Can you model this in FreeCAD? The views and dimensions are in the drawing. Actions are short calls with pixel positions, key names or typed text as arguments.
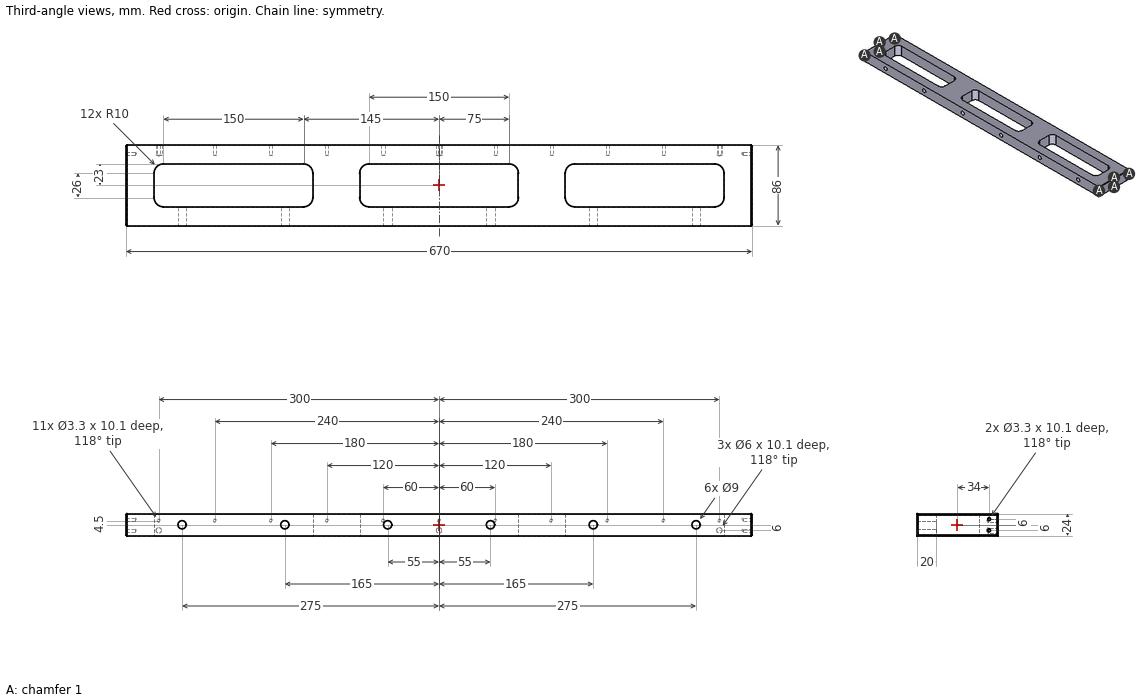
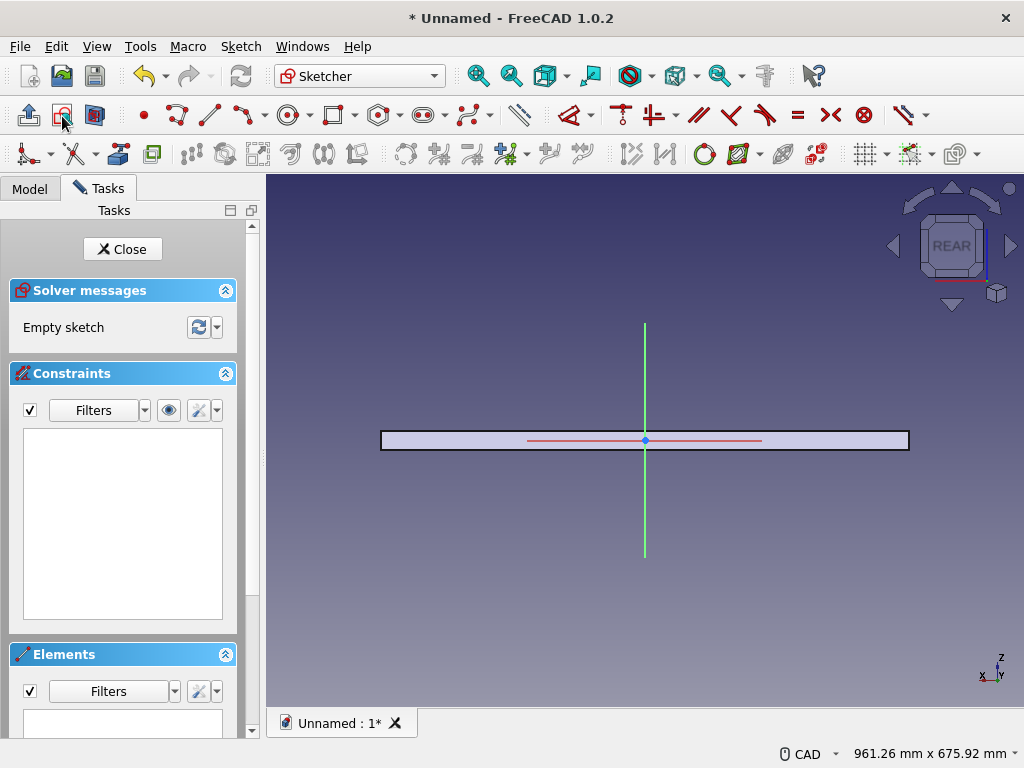
scroll(294, 451, down, 1)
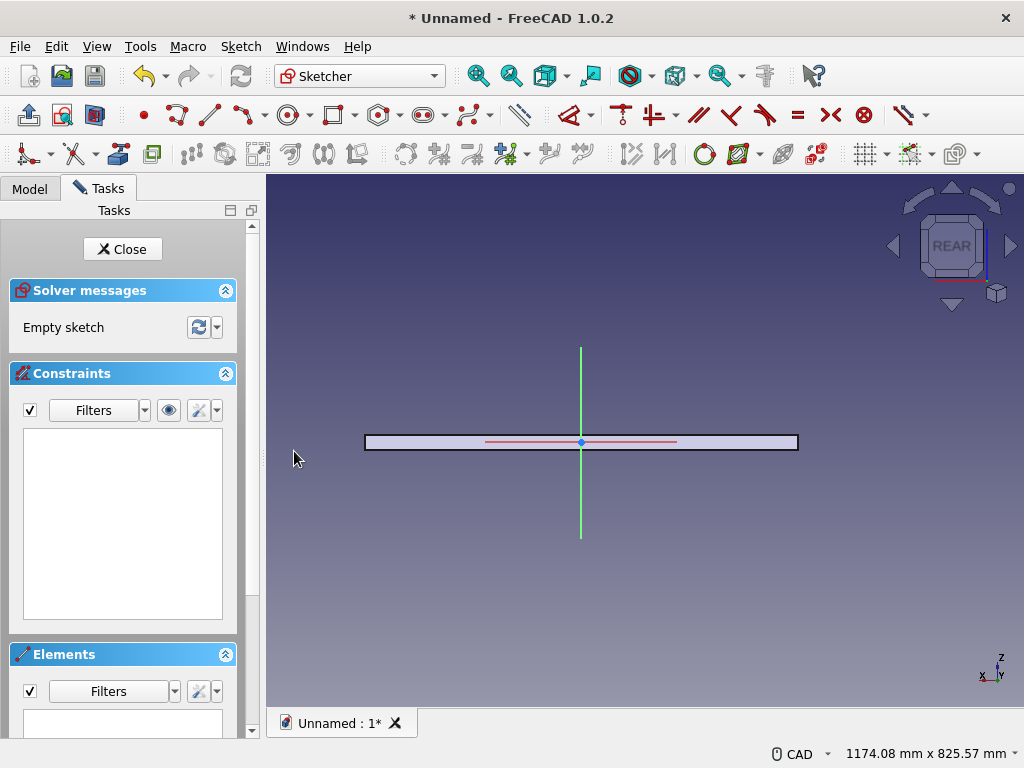
key(g)
key(c)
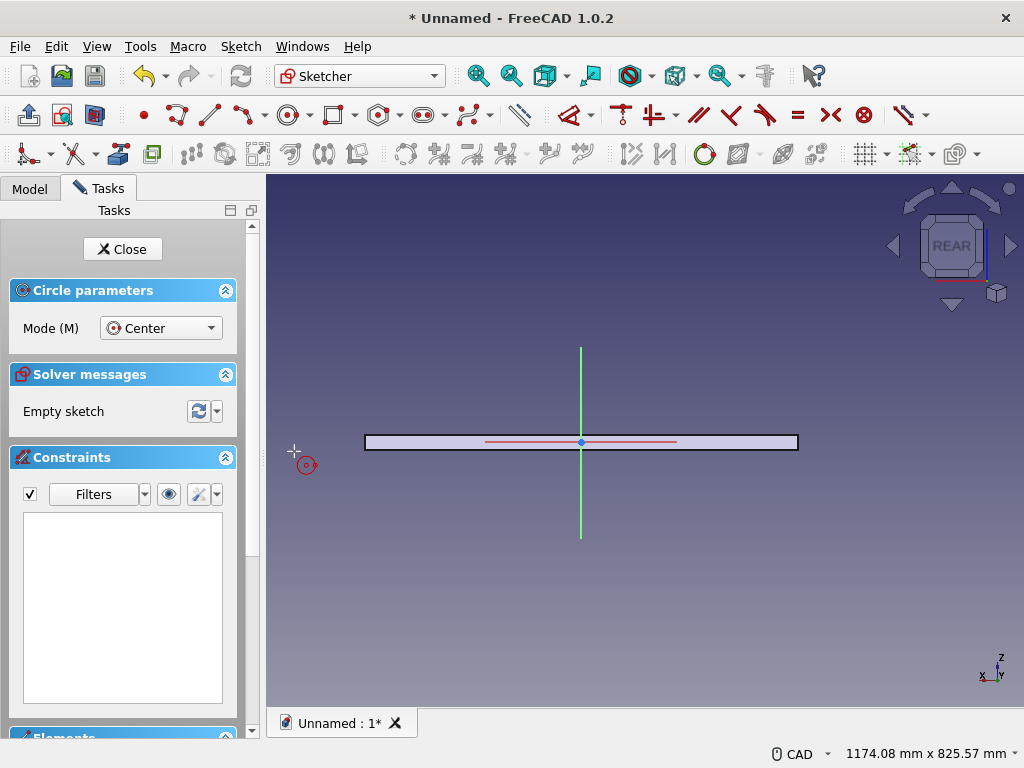
scroll(775, 440, up, 16)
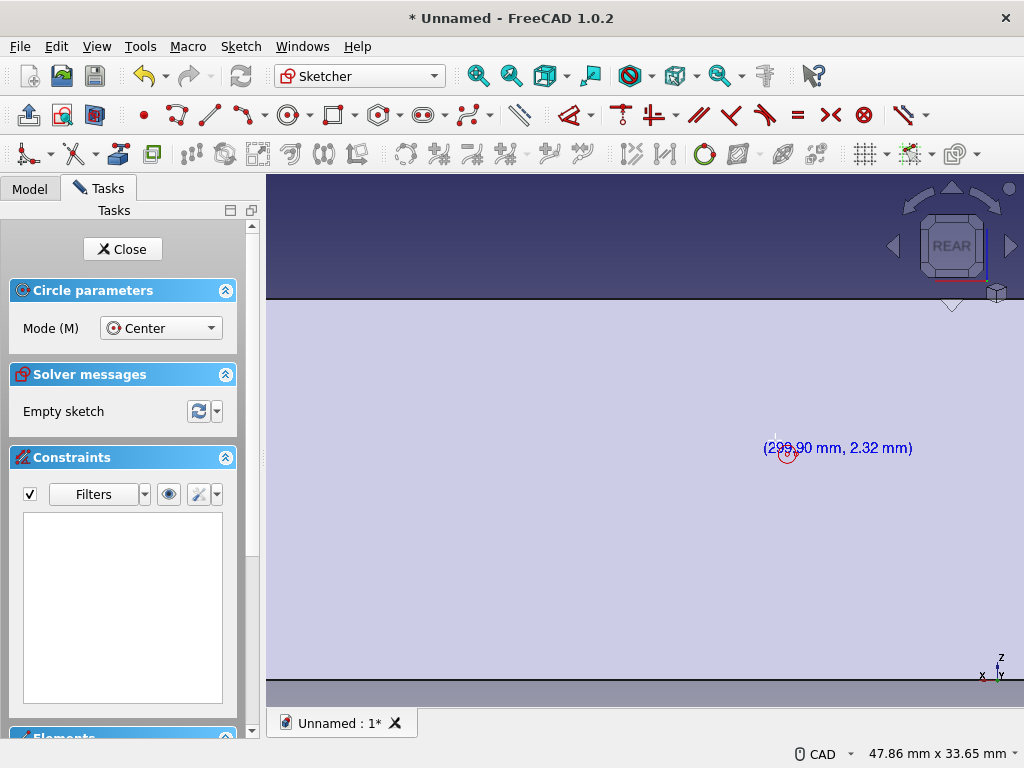
scroll(816, 440, down, 15)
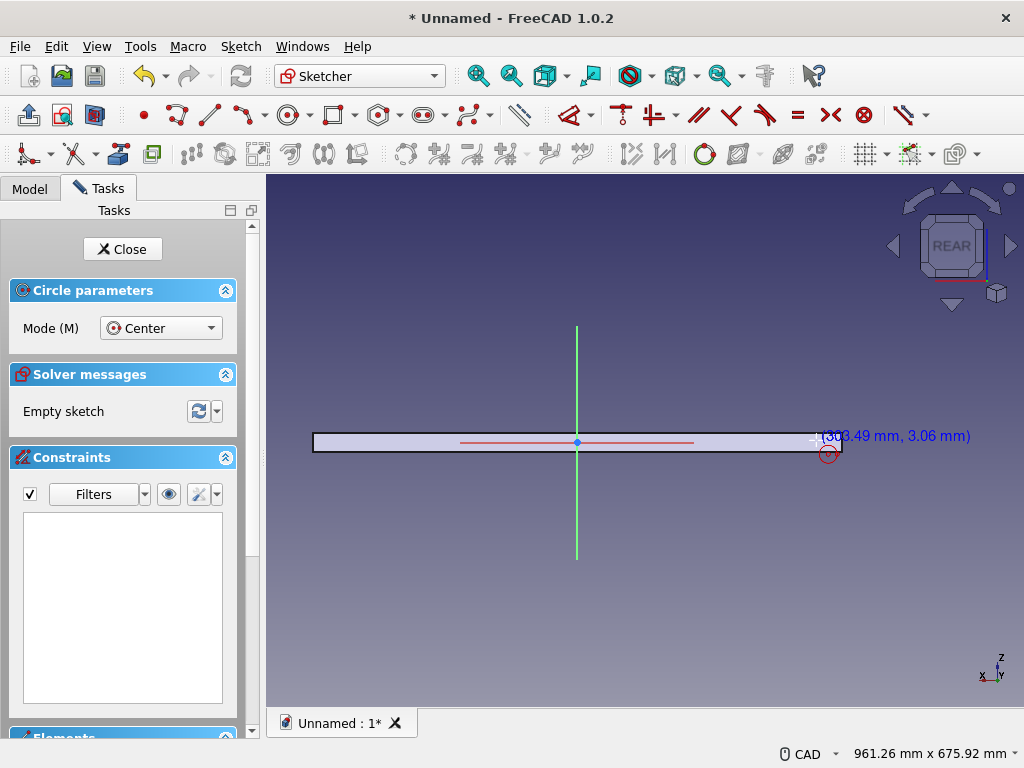
scroll(814, 439, up, 8)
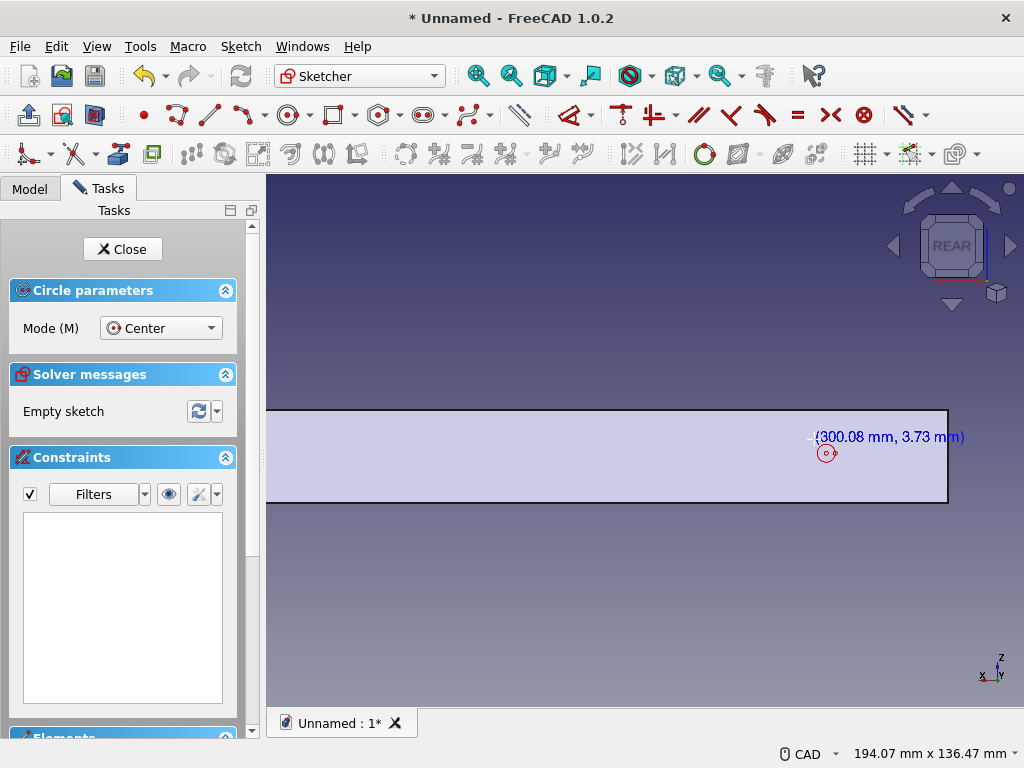
click(811, 439)
move(815, 434)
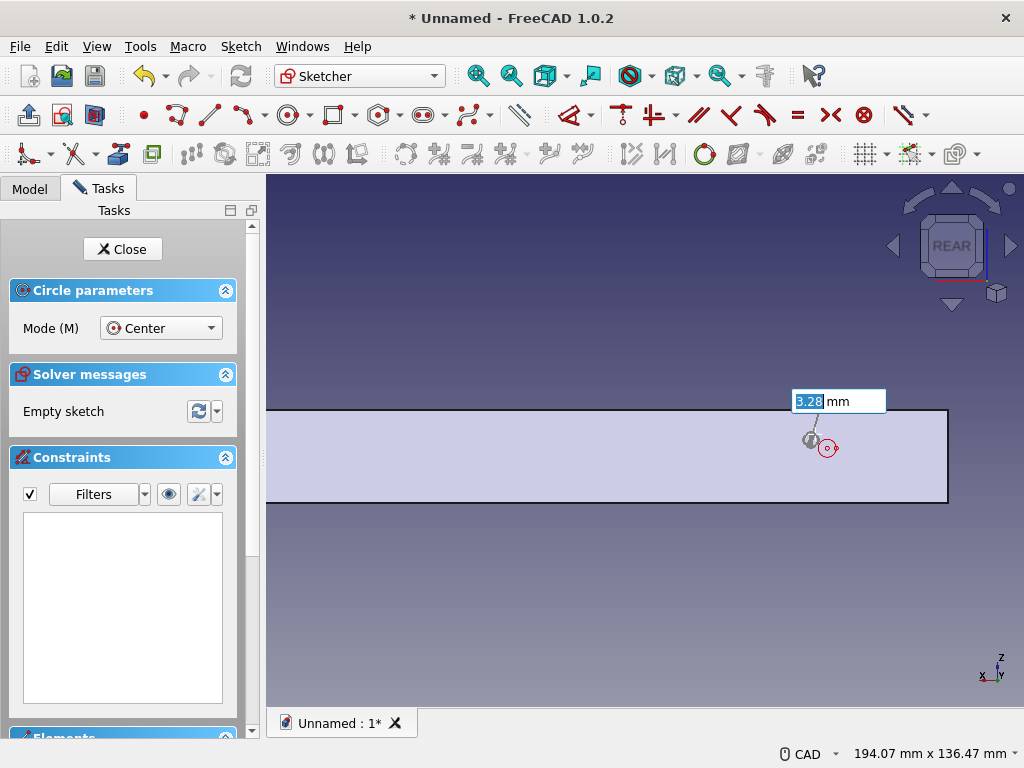
text(3.3)
key(Return)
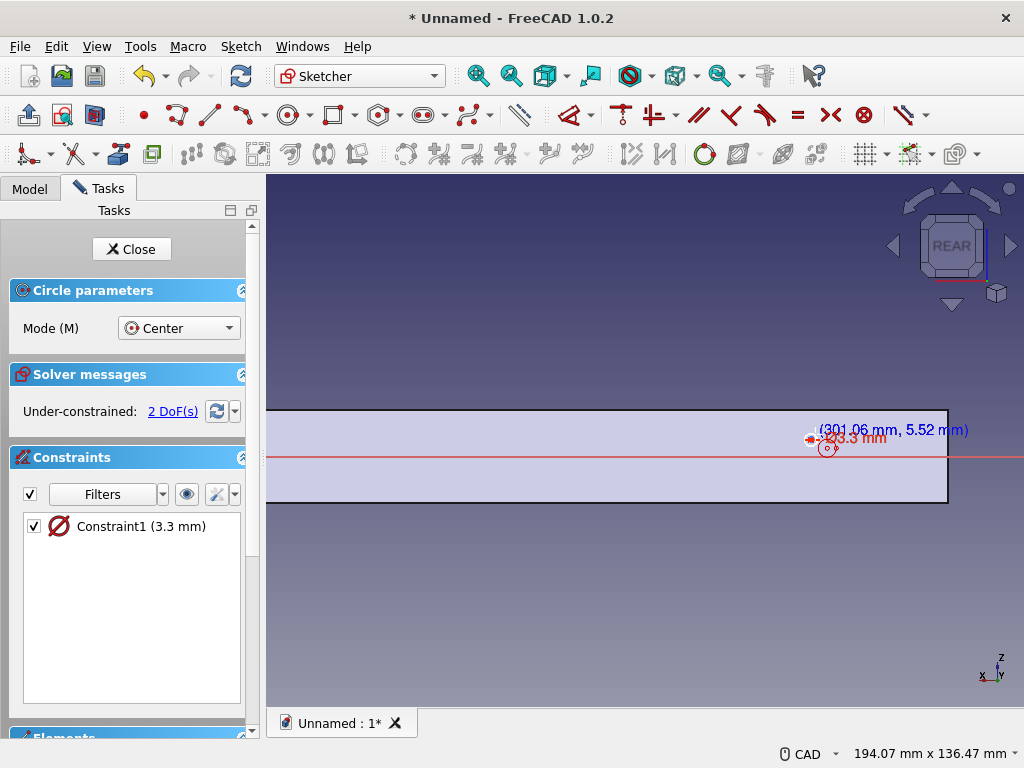
scroll(576, 439, up, 7)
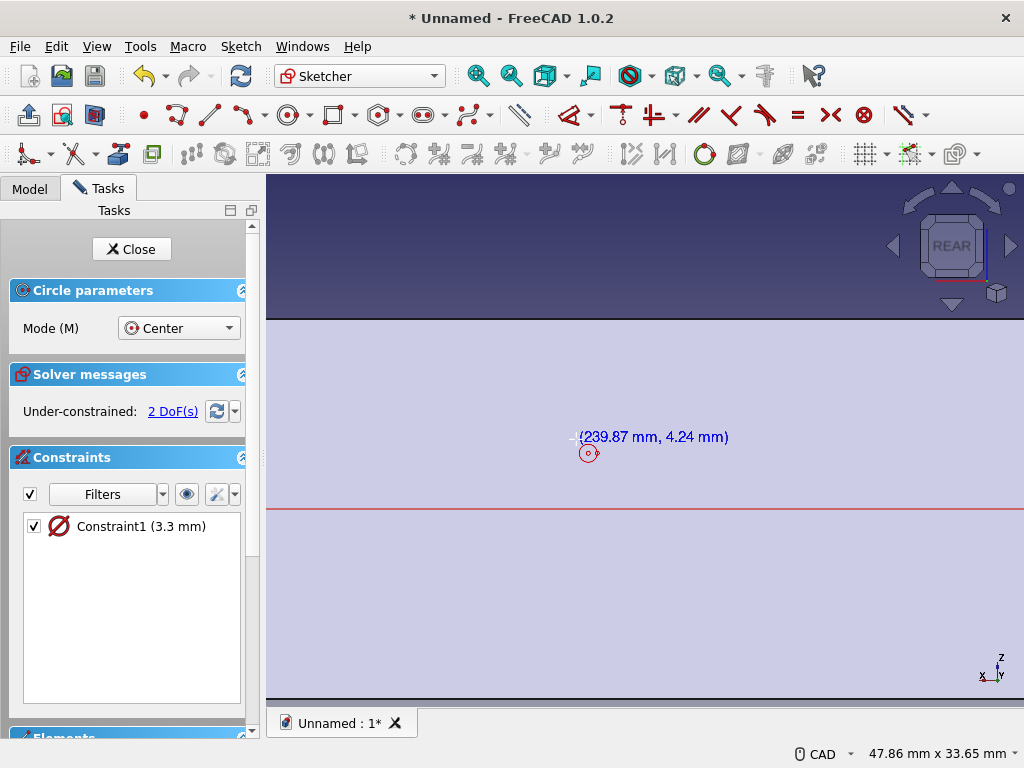
scroll(776, 439, down, 15)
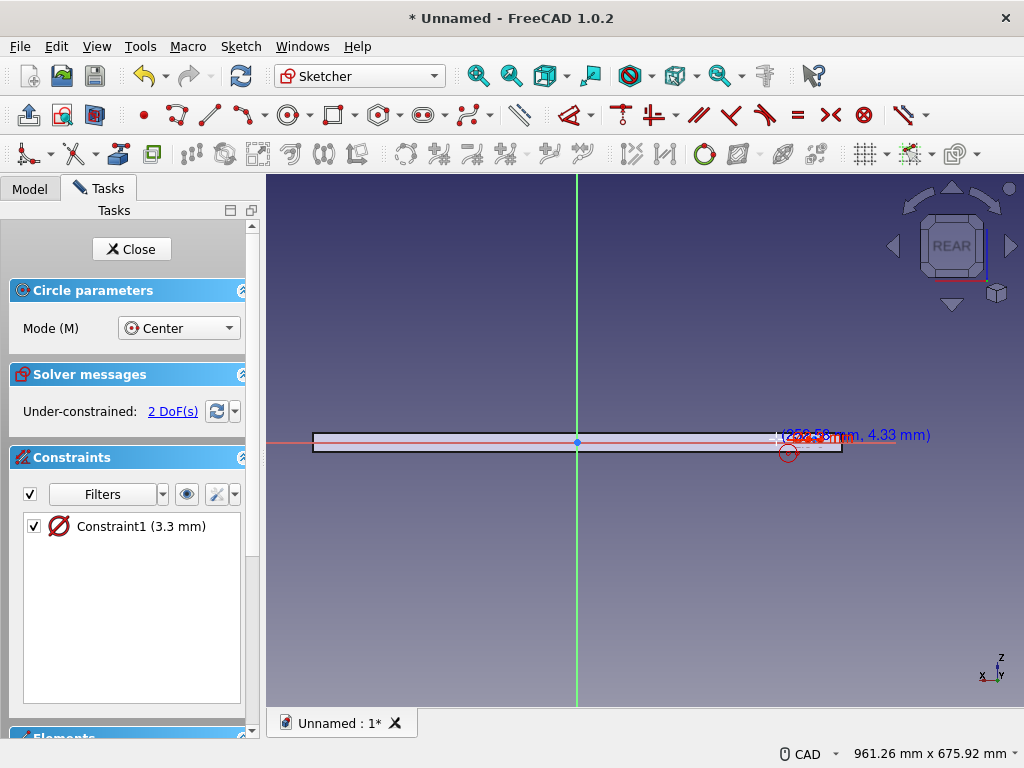
scroll(767, 439, up, 8)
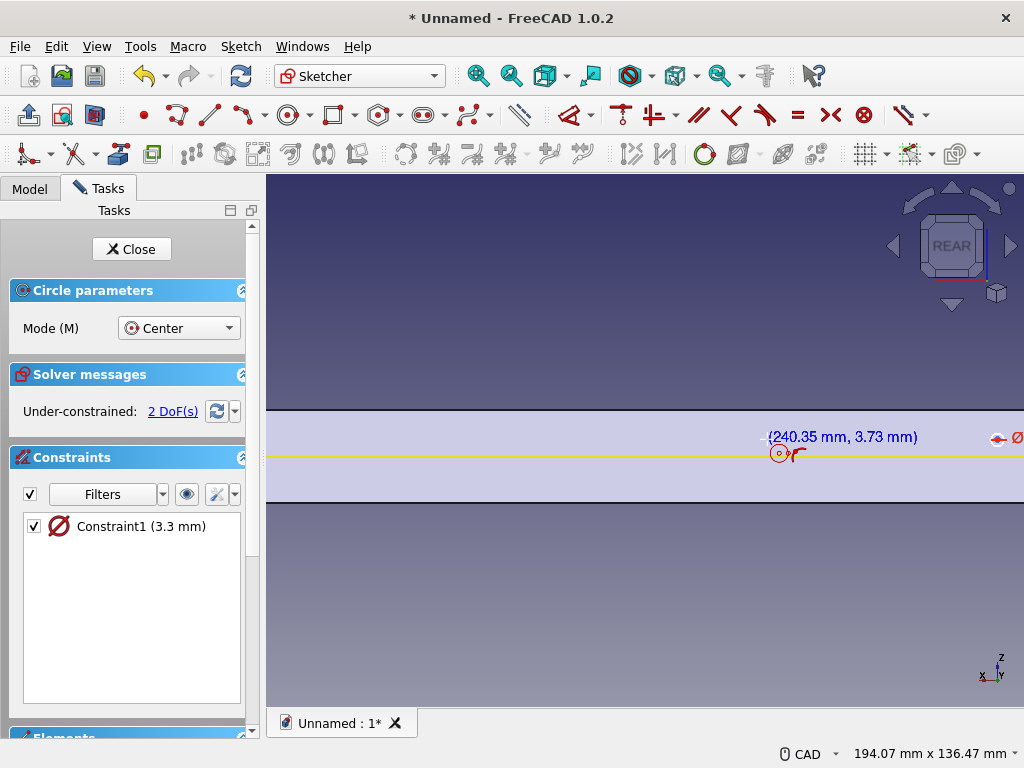
click(763, 439)
move(768, 434)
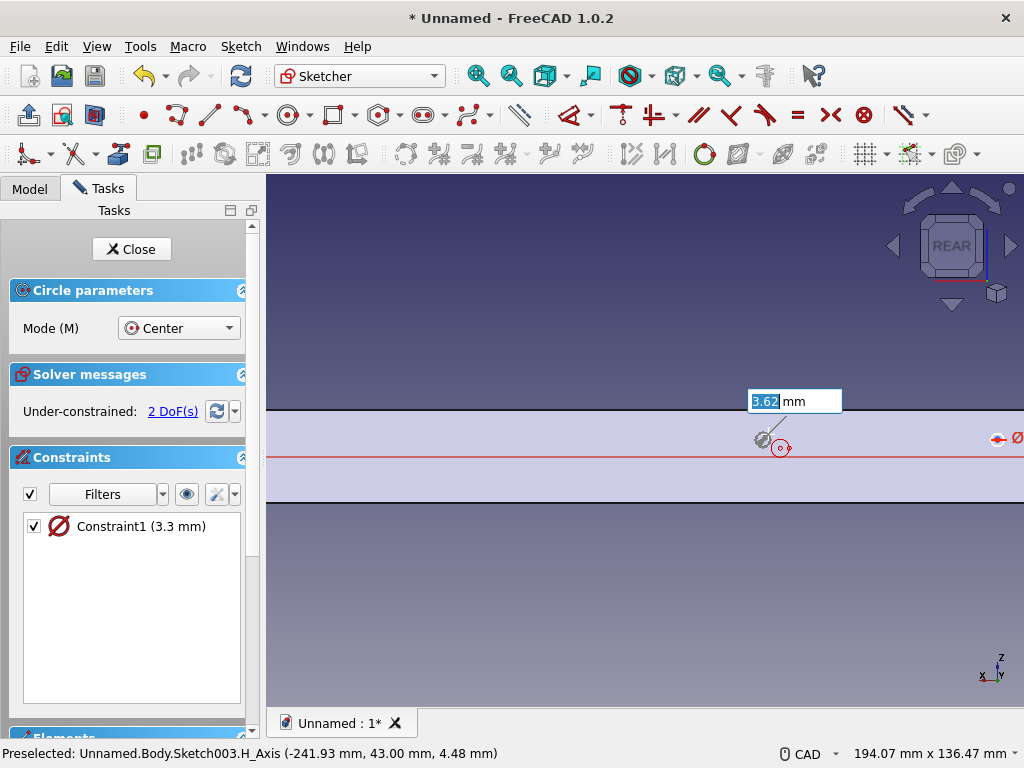
text(3.3)
key(Return)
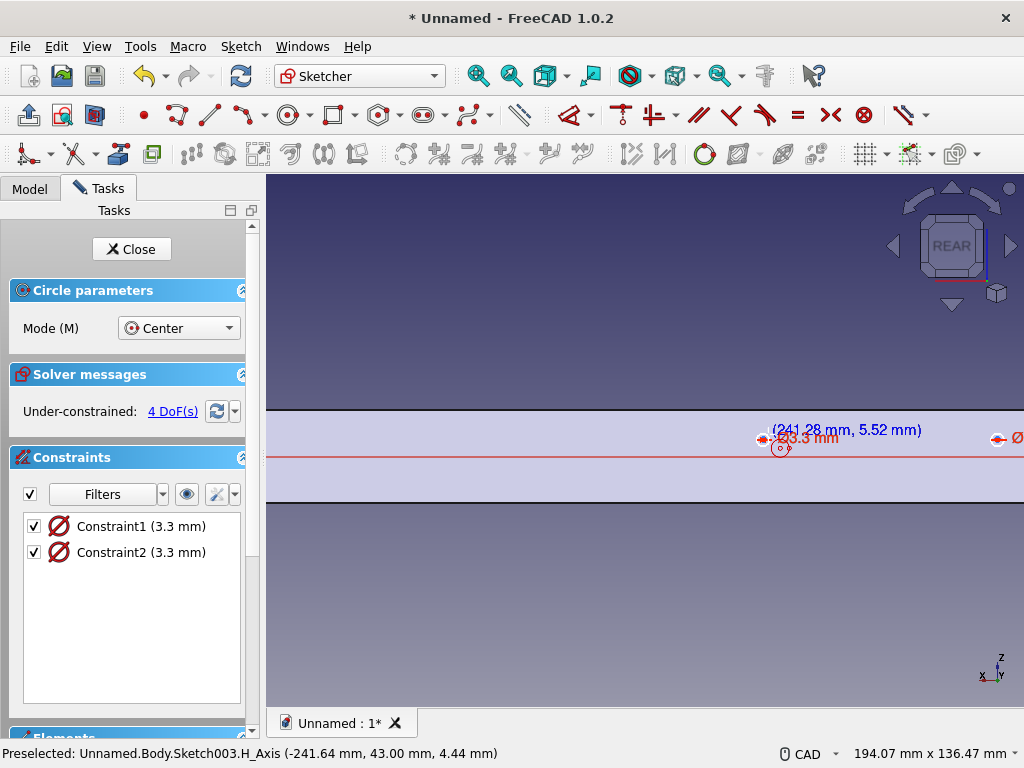
scroll(529, 439, up, 7)